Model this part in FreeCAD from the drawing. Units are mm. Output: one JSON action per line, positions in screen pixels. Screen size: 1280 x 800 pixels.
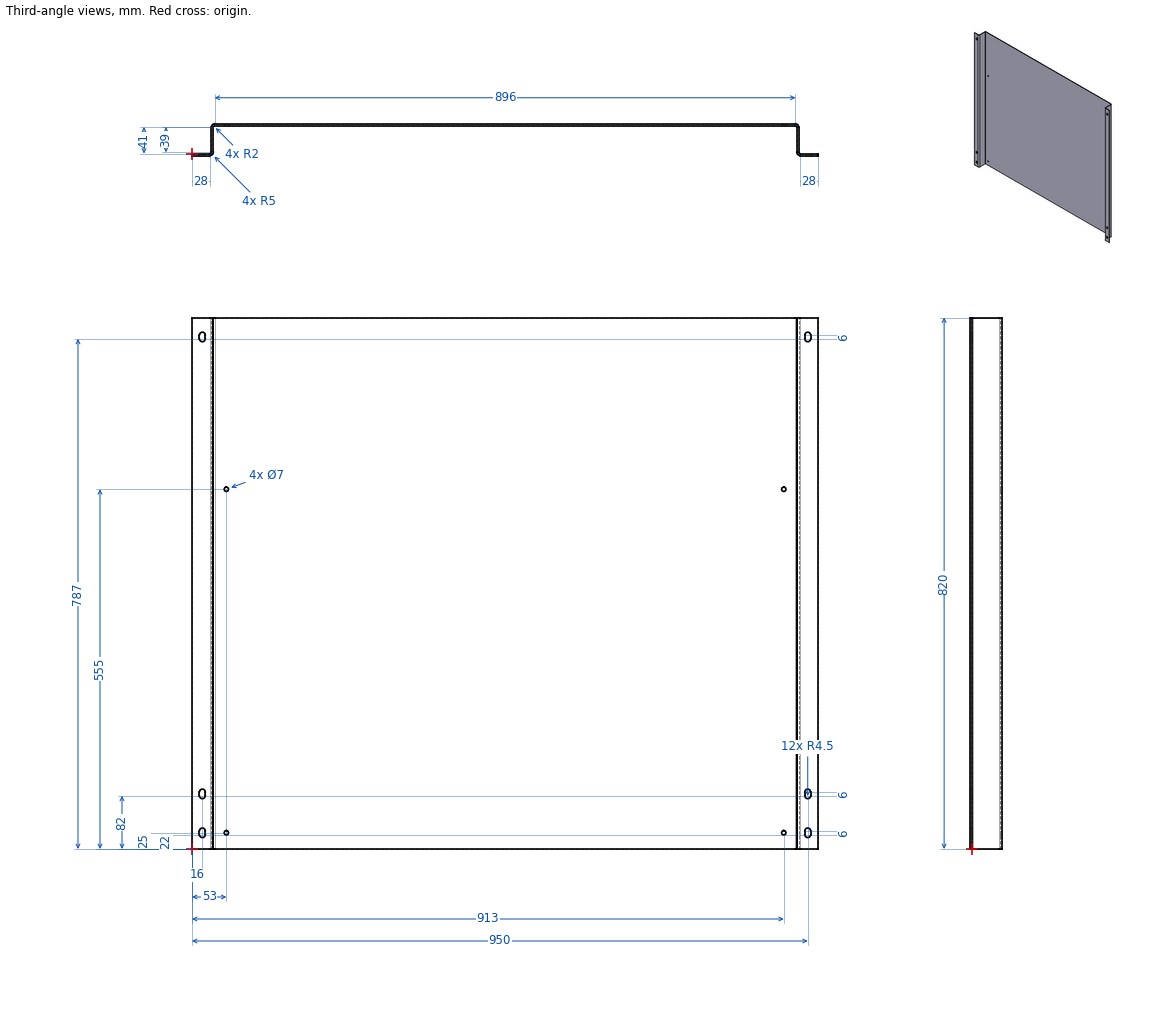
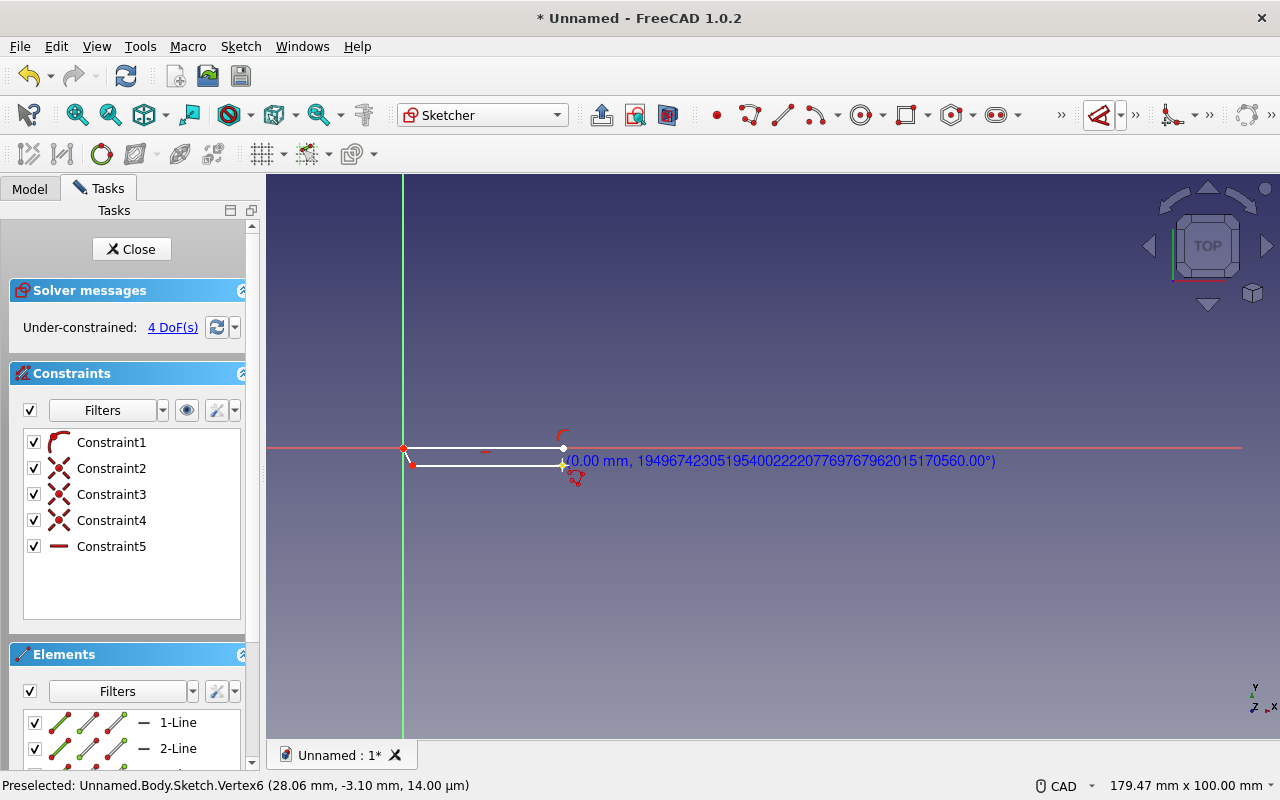
{"action": "key", "text": "g l"}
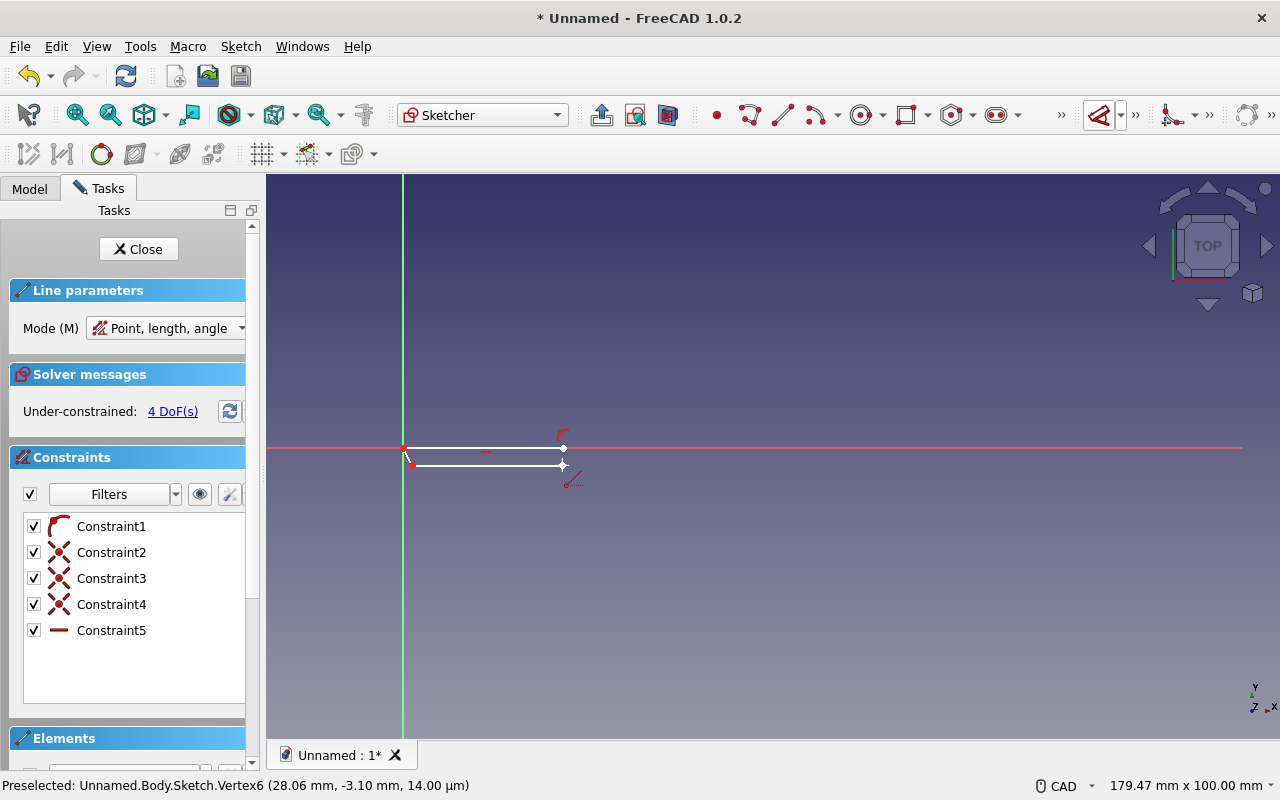
{"action": "scroll", "coordinate": [590, 437], "scroll_direction": "up", "scroll_amount": 2}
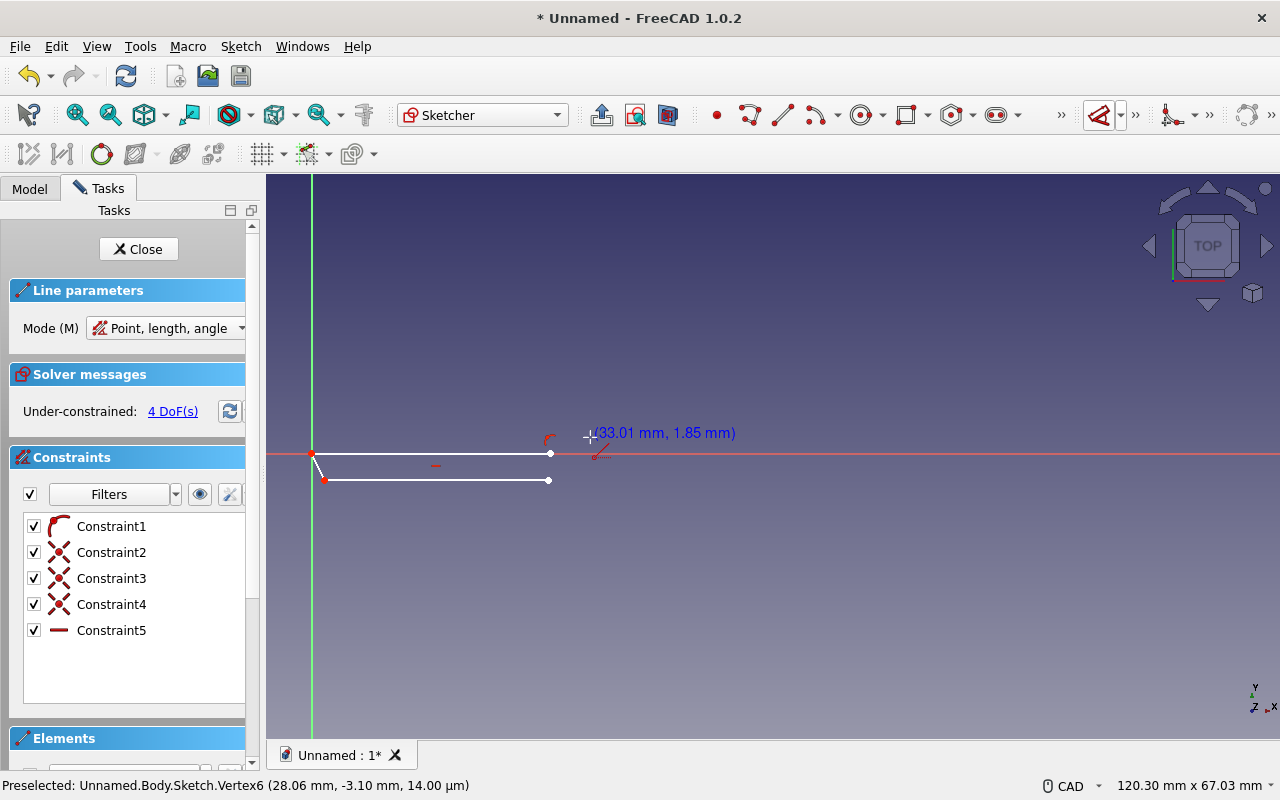
{"action": "left_click", "coordinate": [590, 437]}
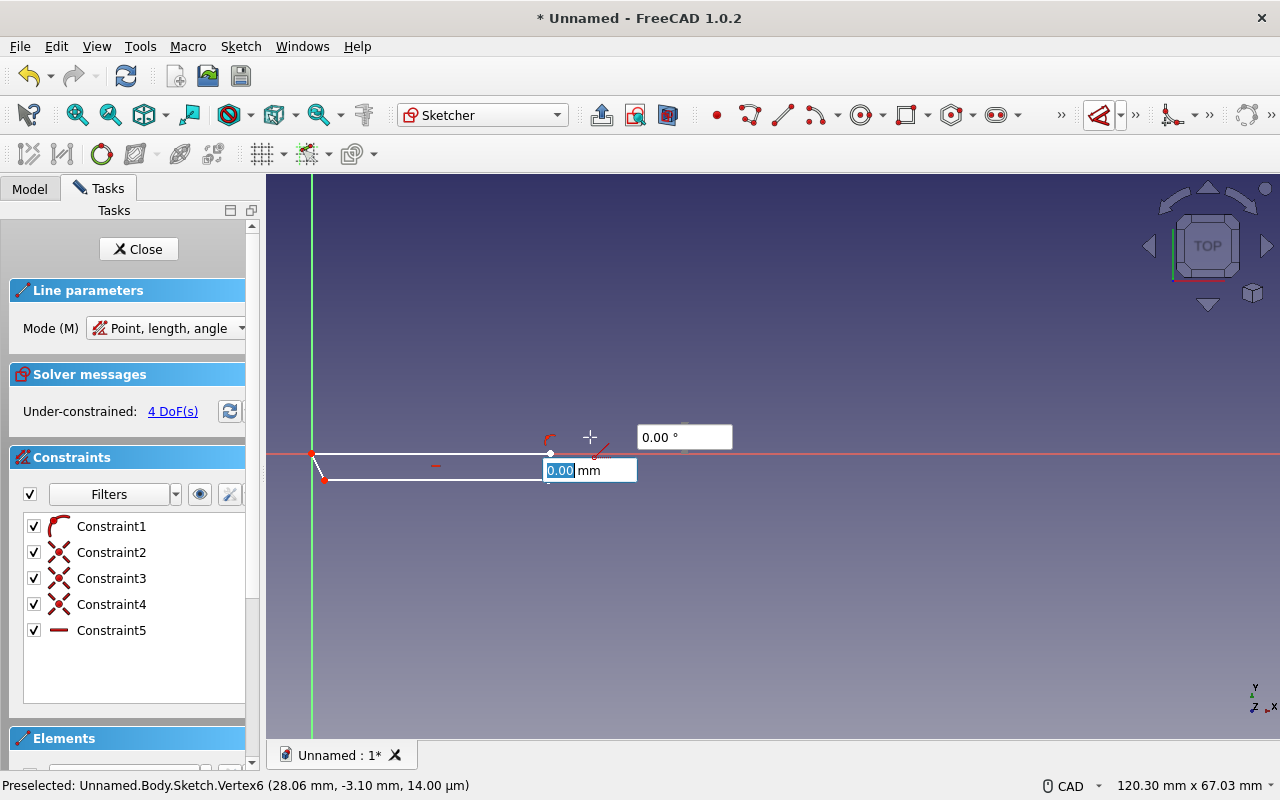
{"action": "scroll", "coordinate": [409, 471], "scroll_direction": "down", "scroll_amount": 13}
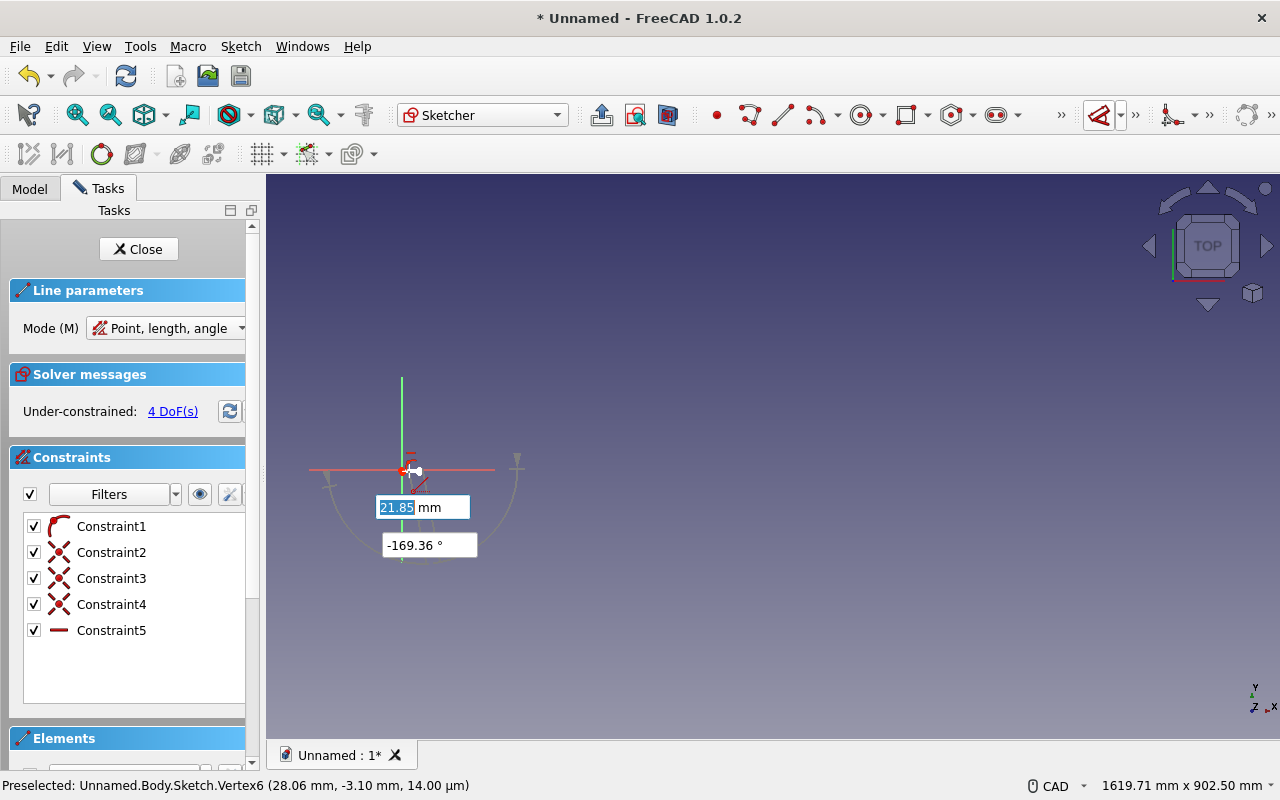
{"action": "left_click", "coordinate": [423, 445]}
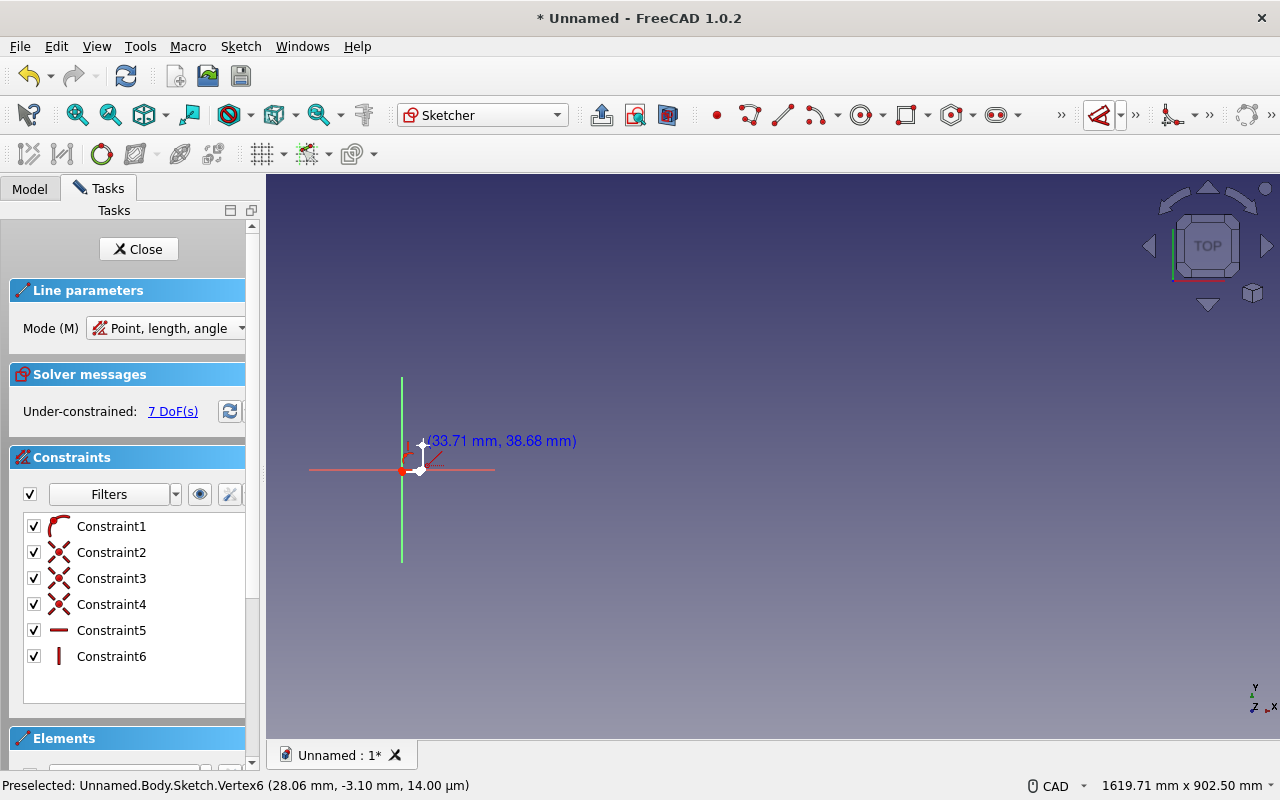
{"action": "scroll", "coordinate": [424, 443], "scroll_direction": "up", "scroll_amount": 11}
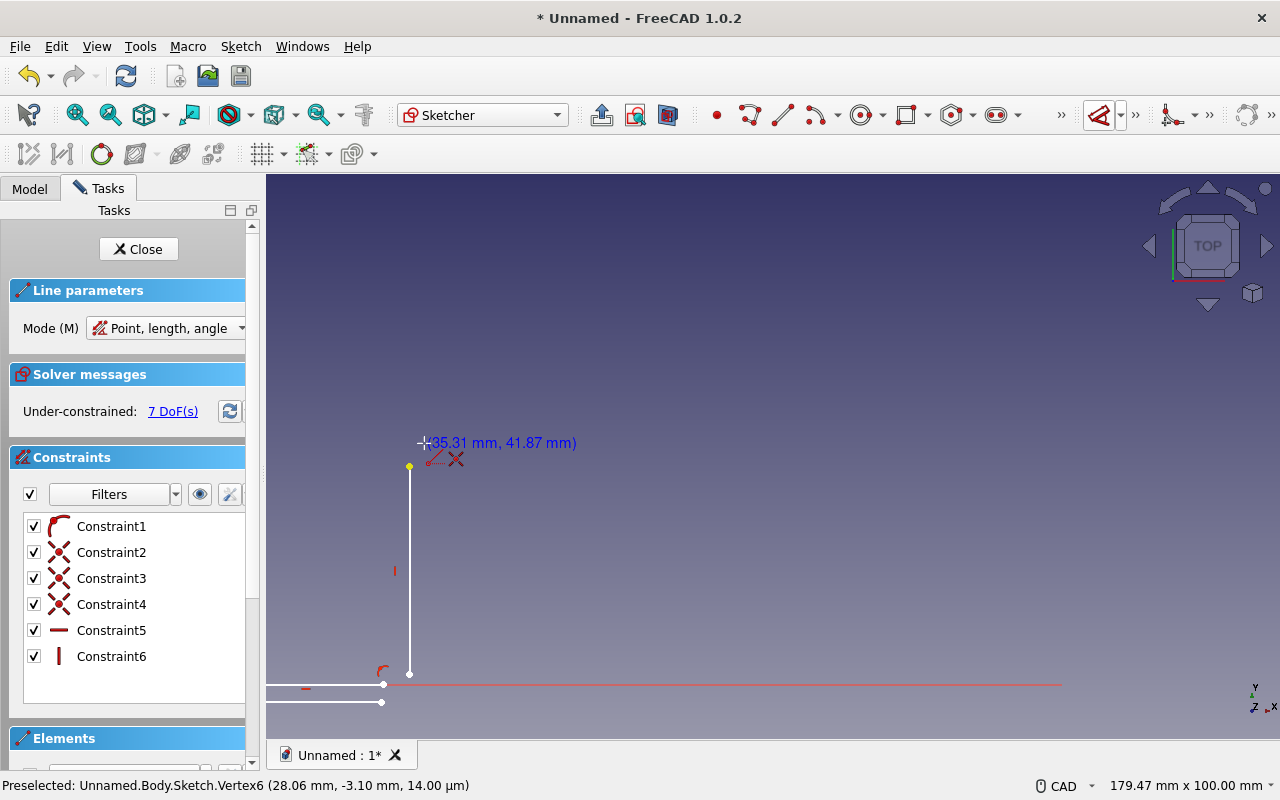
{"action": "left_click", "coordinate": [421, 442]}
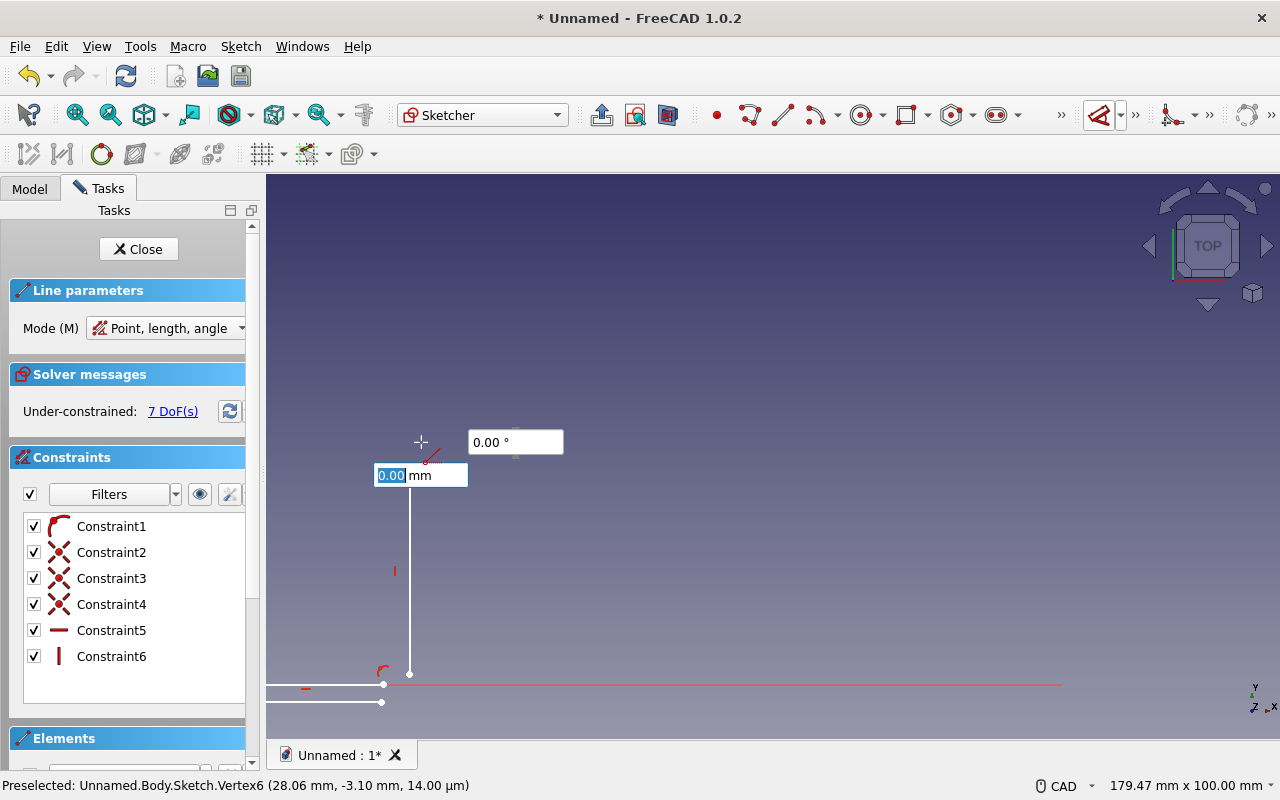
{"action": "scroll", "coordinate": [424, 443], "scroll_direction": "down", "scroll_amount": 11}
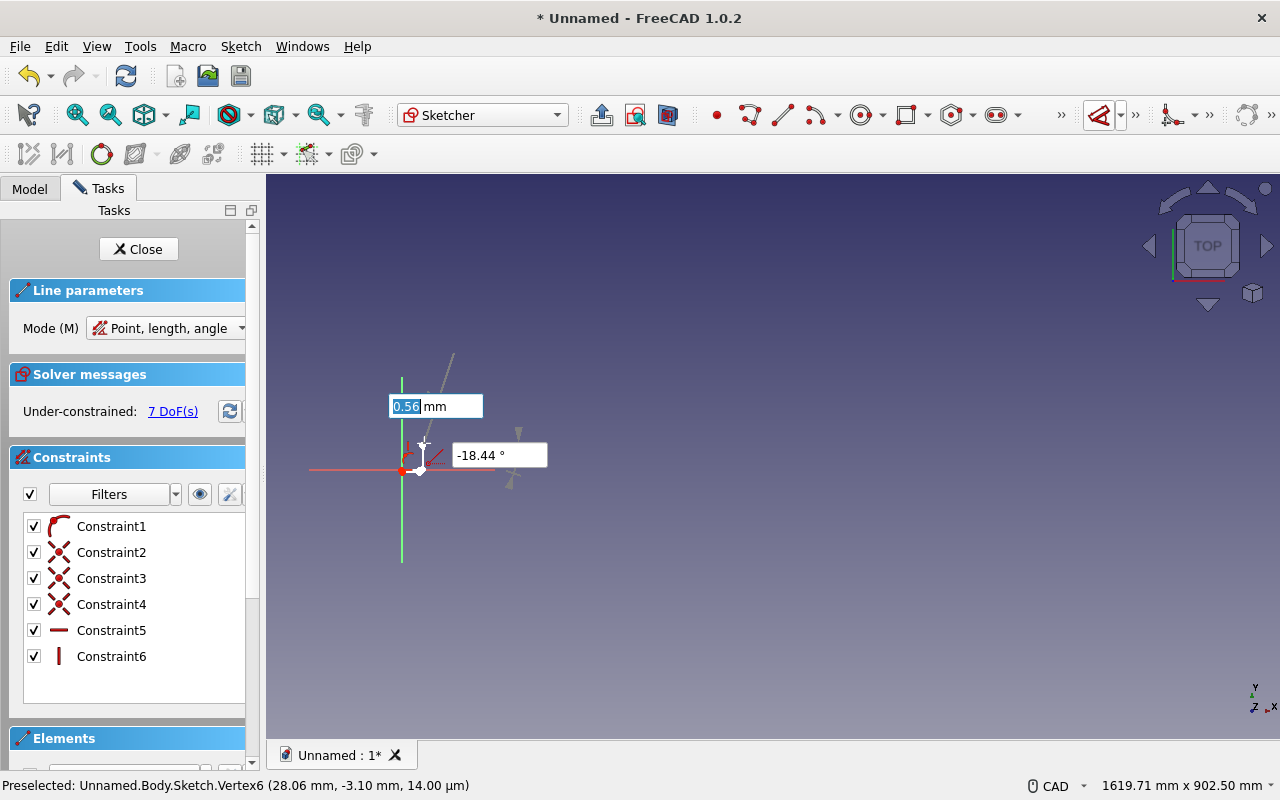
{"action": "left_click", "coordinate": [985, 443]}